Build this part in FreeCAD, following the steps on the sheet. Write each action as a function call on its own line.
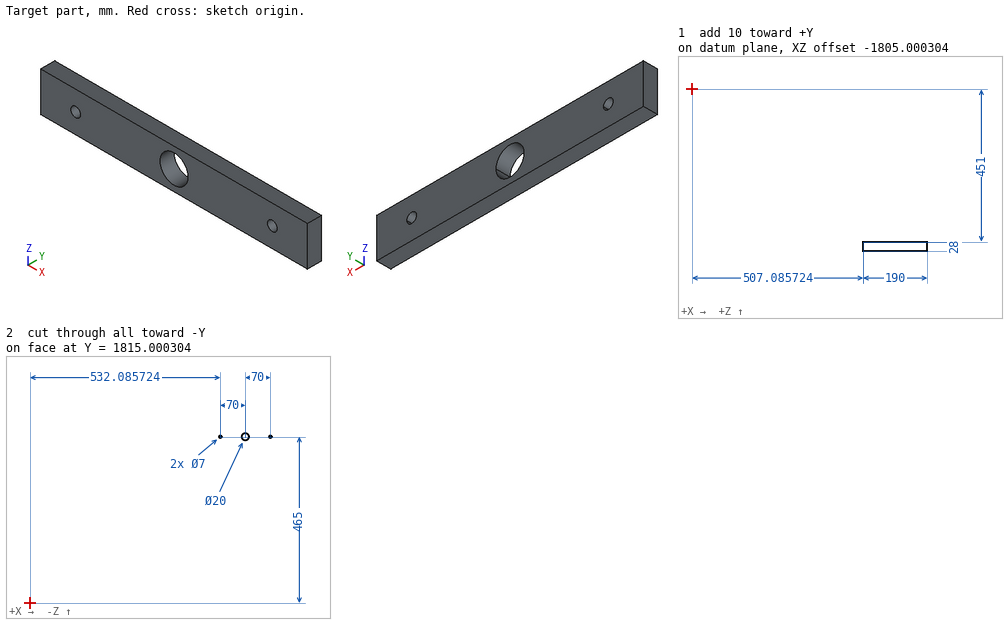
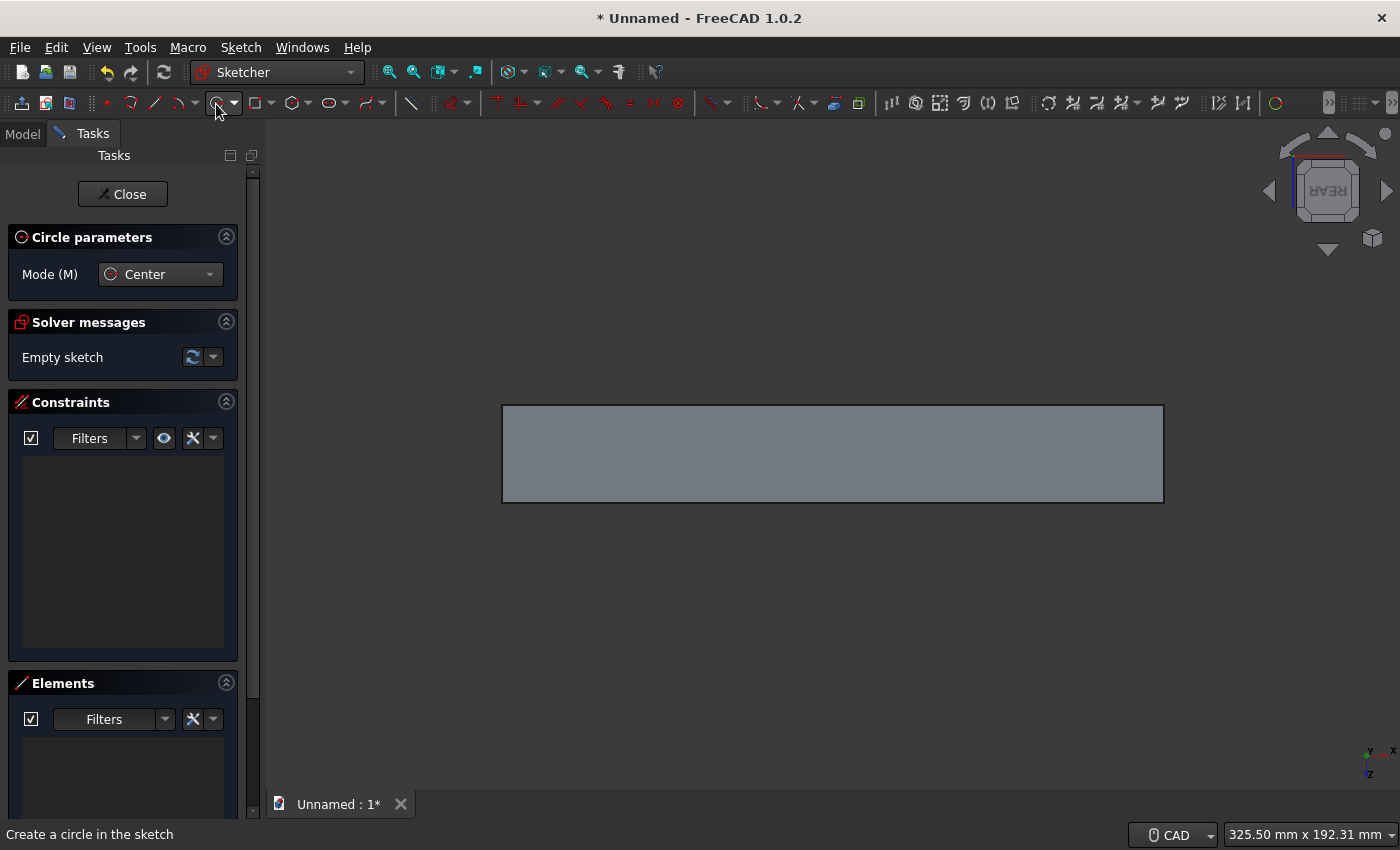
scroll(589, 454, up, 4)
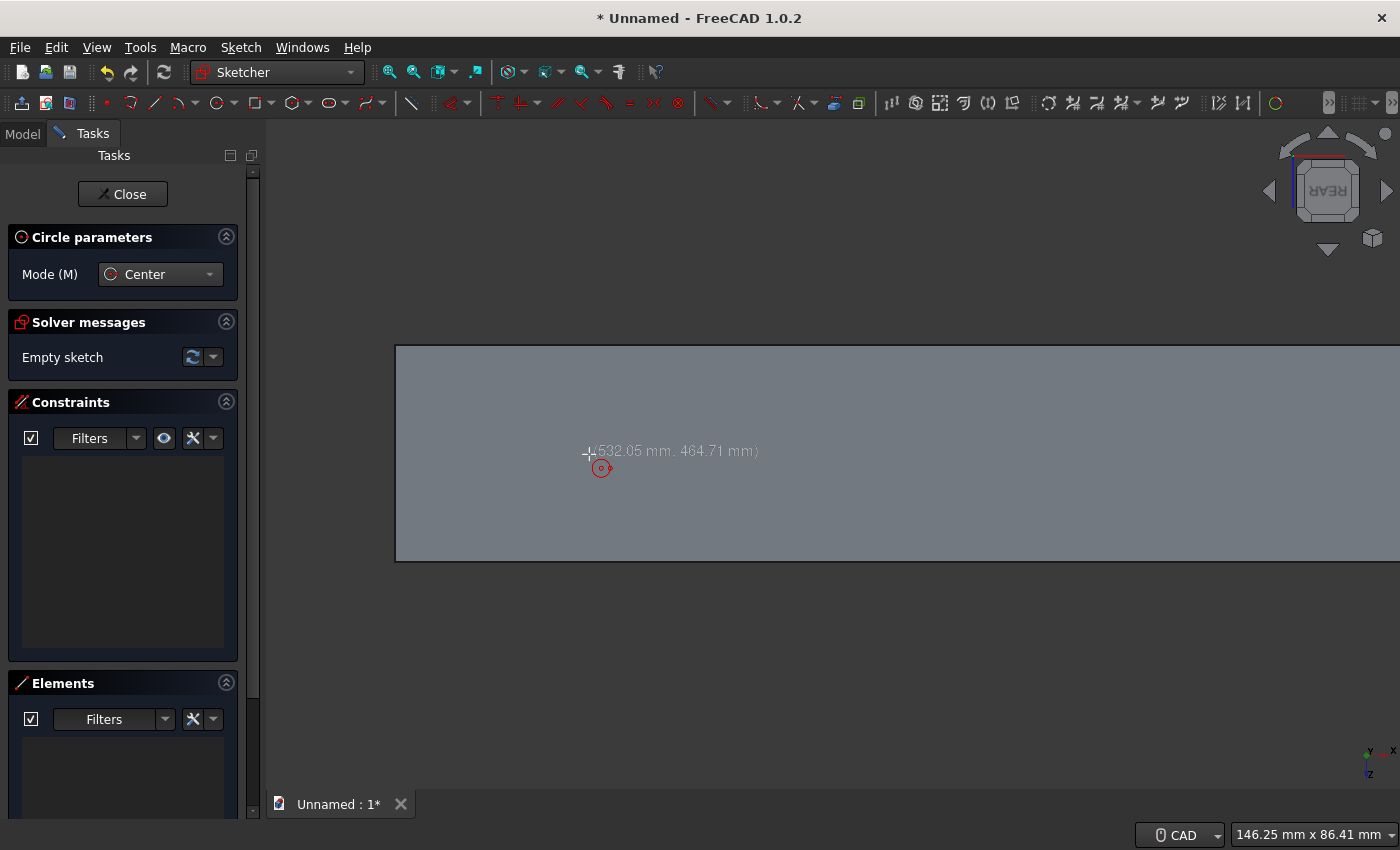
click(589, 453)
click(608, 434)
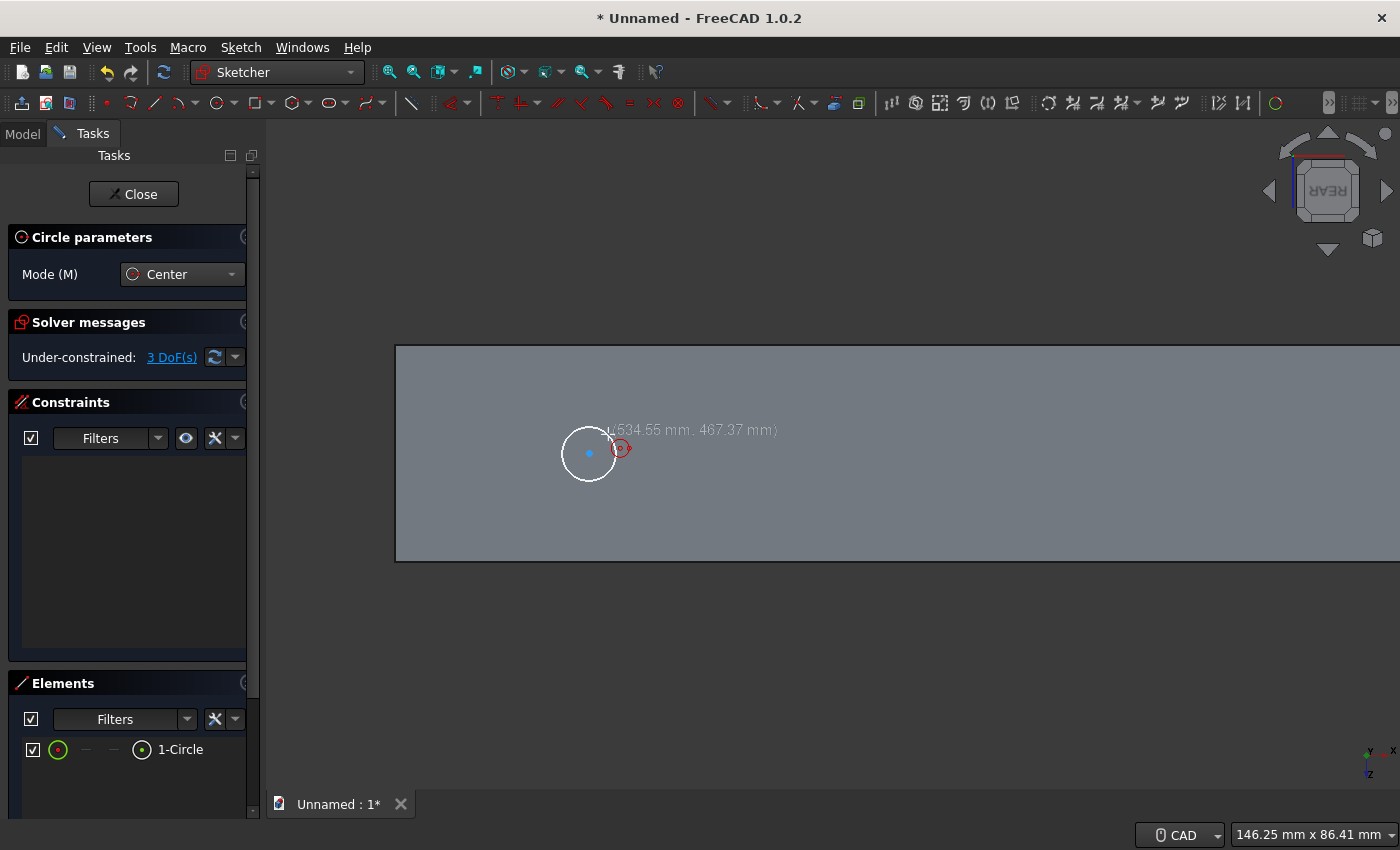
scroll(318, 455, down, 3)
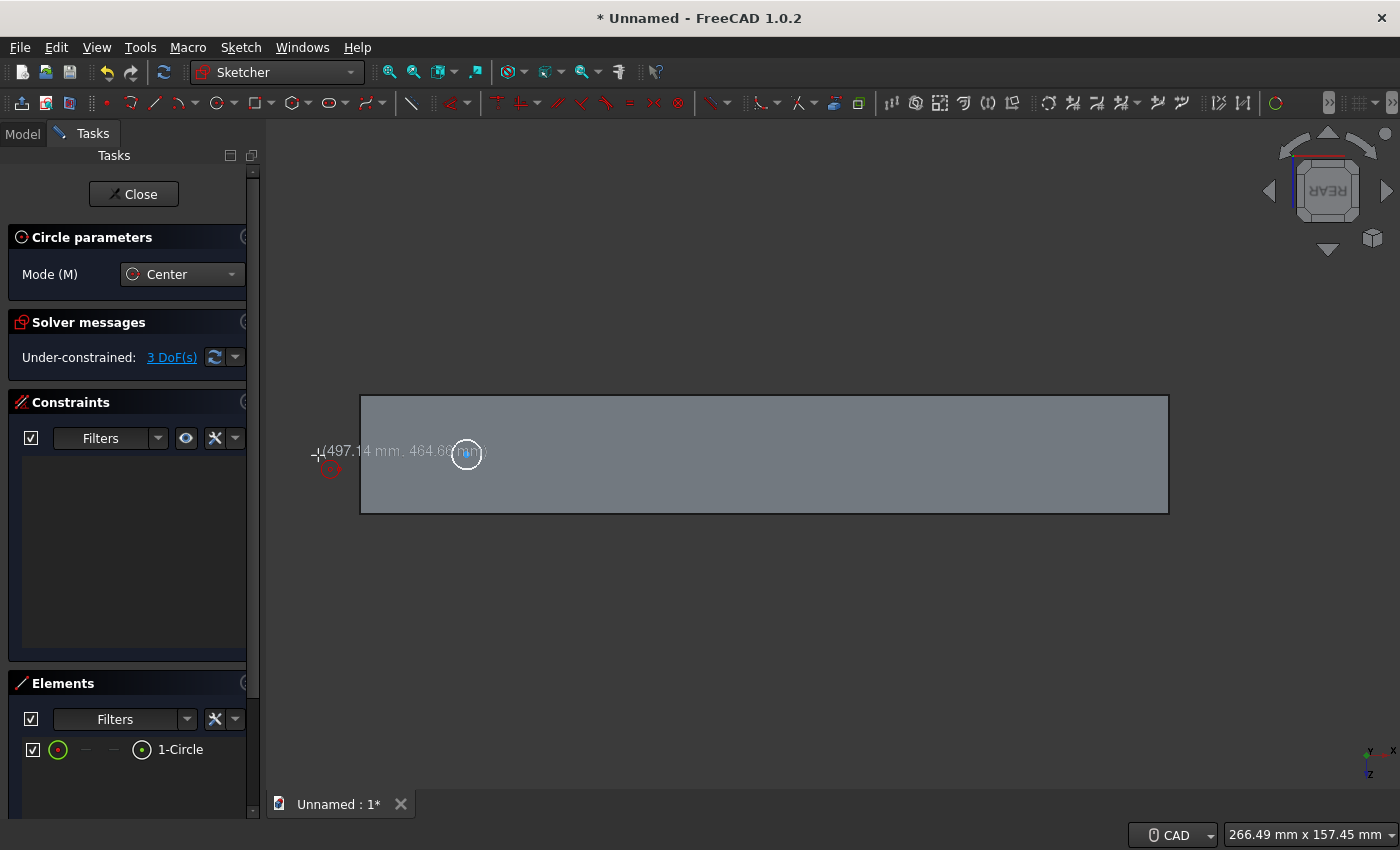
scroll(1062, 454, up, 3)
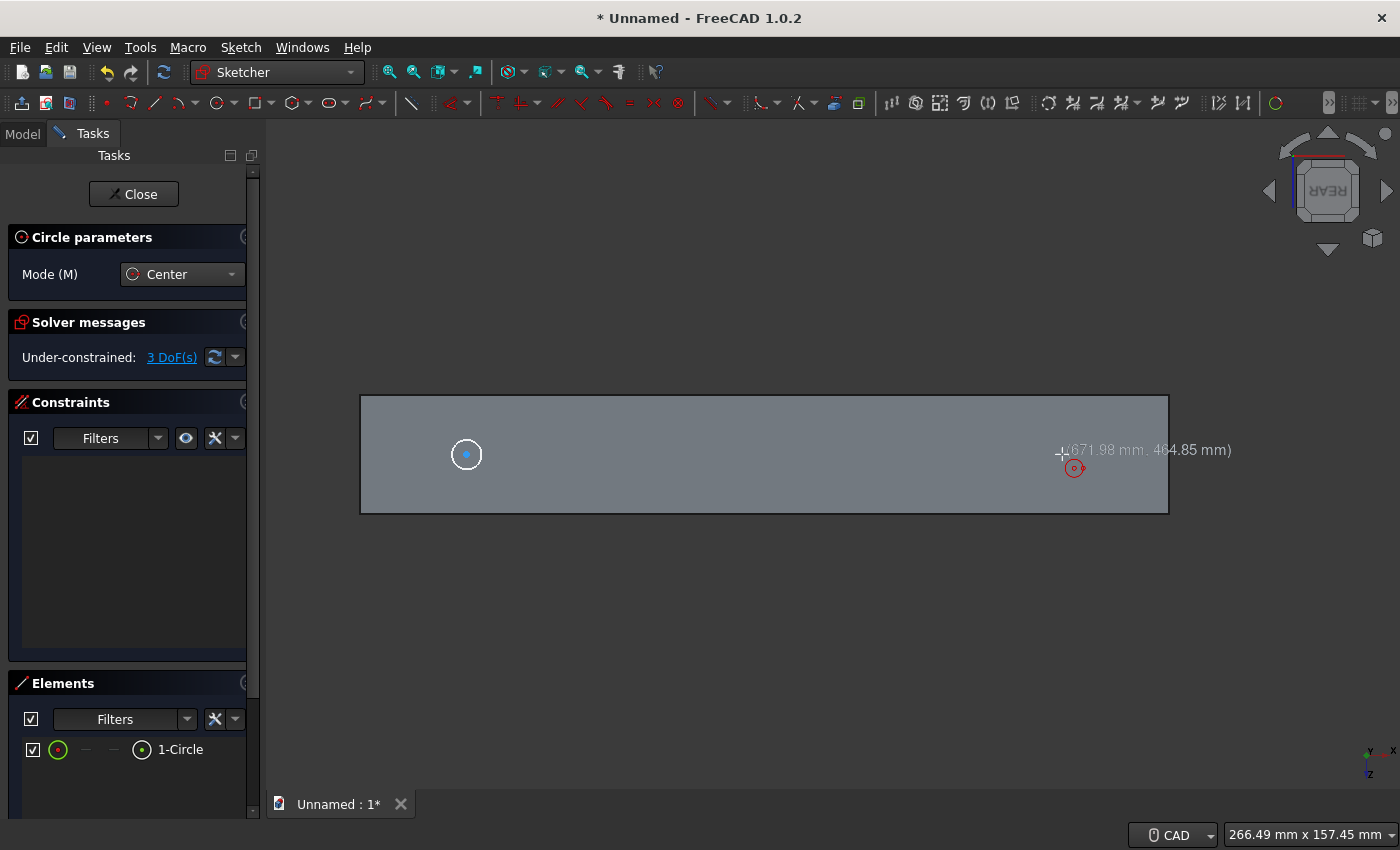
click(1062, 454)
click(1081, 435)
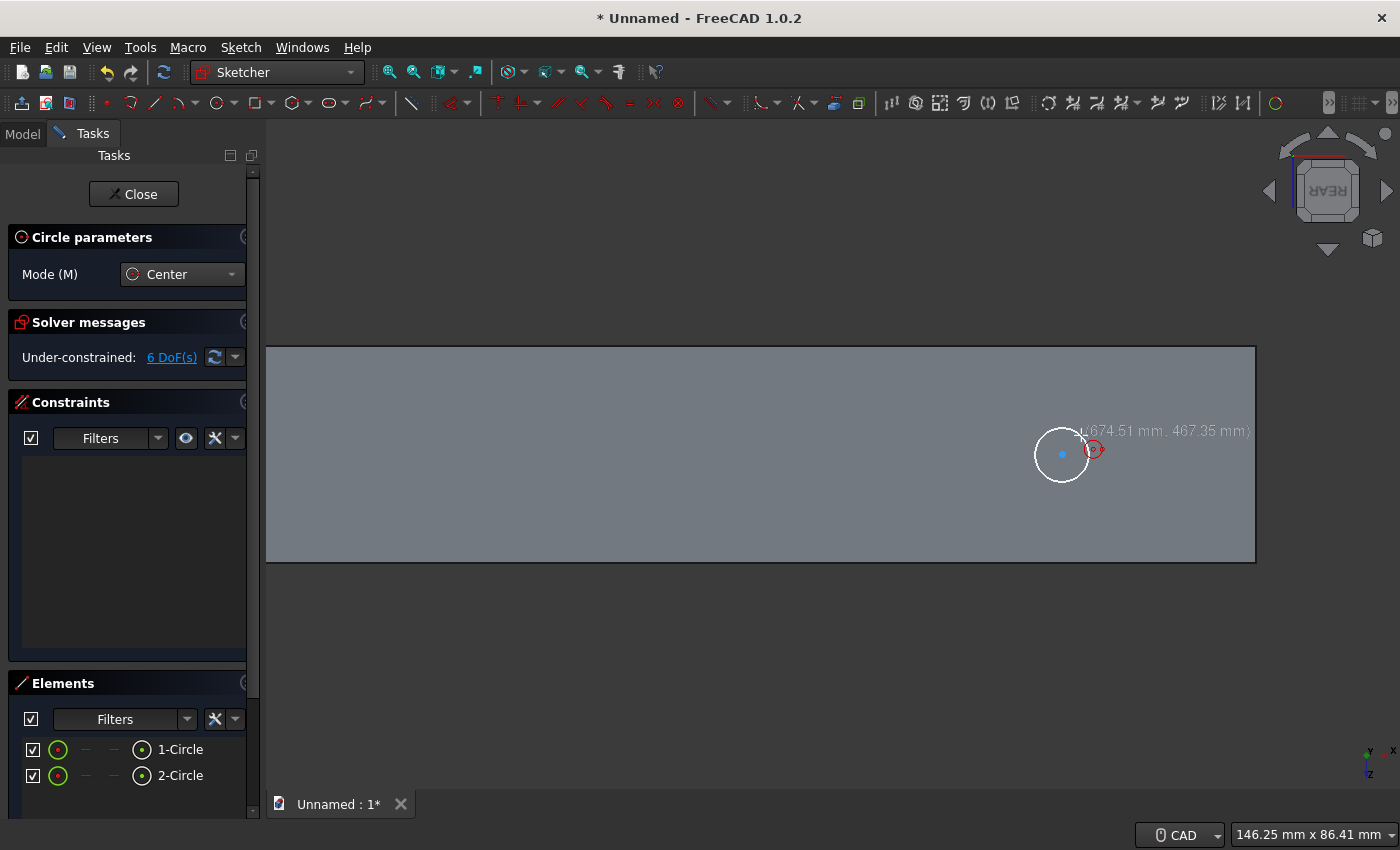
click(519, 454)
click(574, 399)
key(Escape)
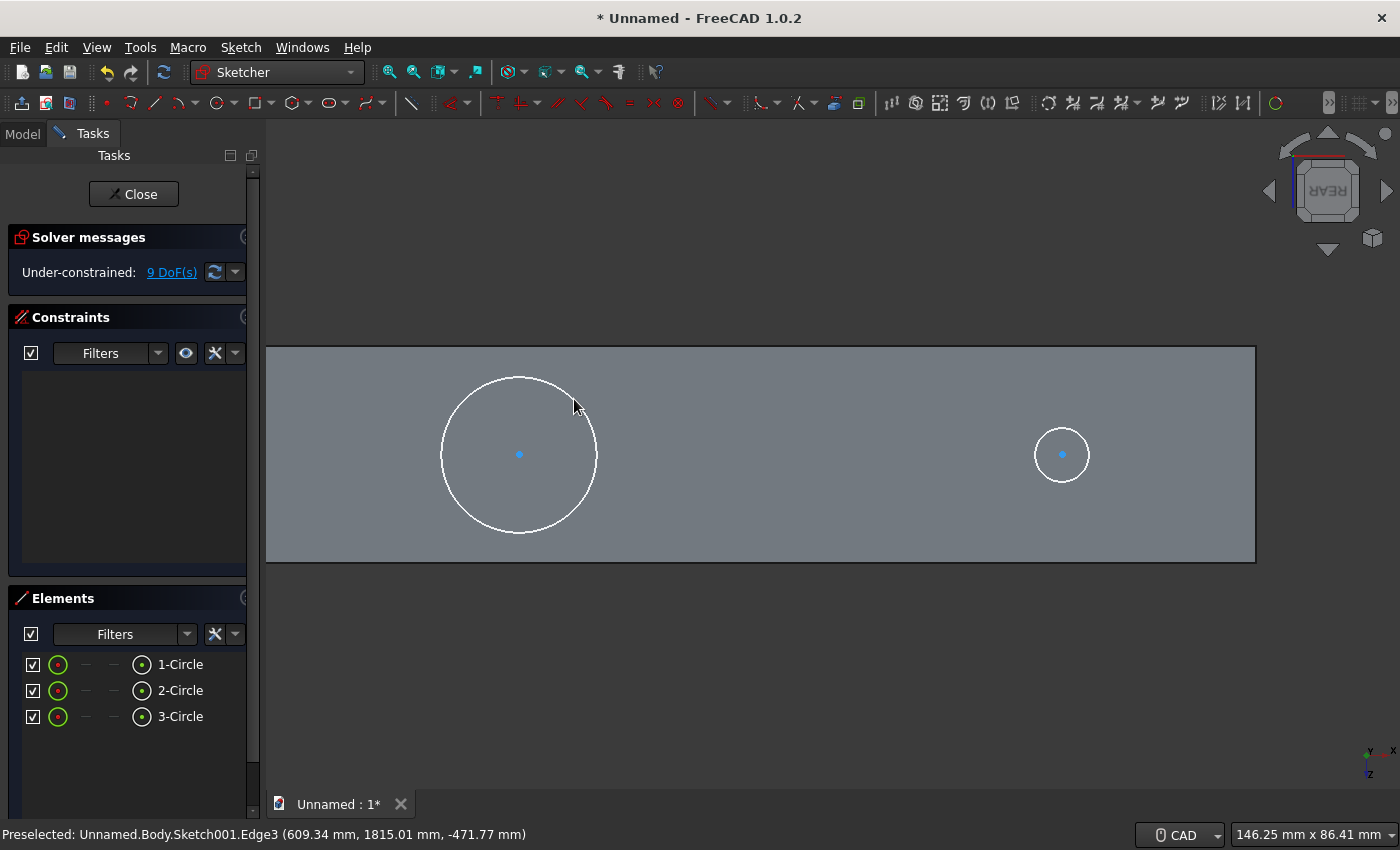
scroll(1063, 454, down, 3)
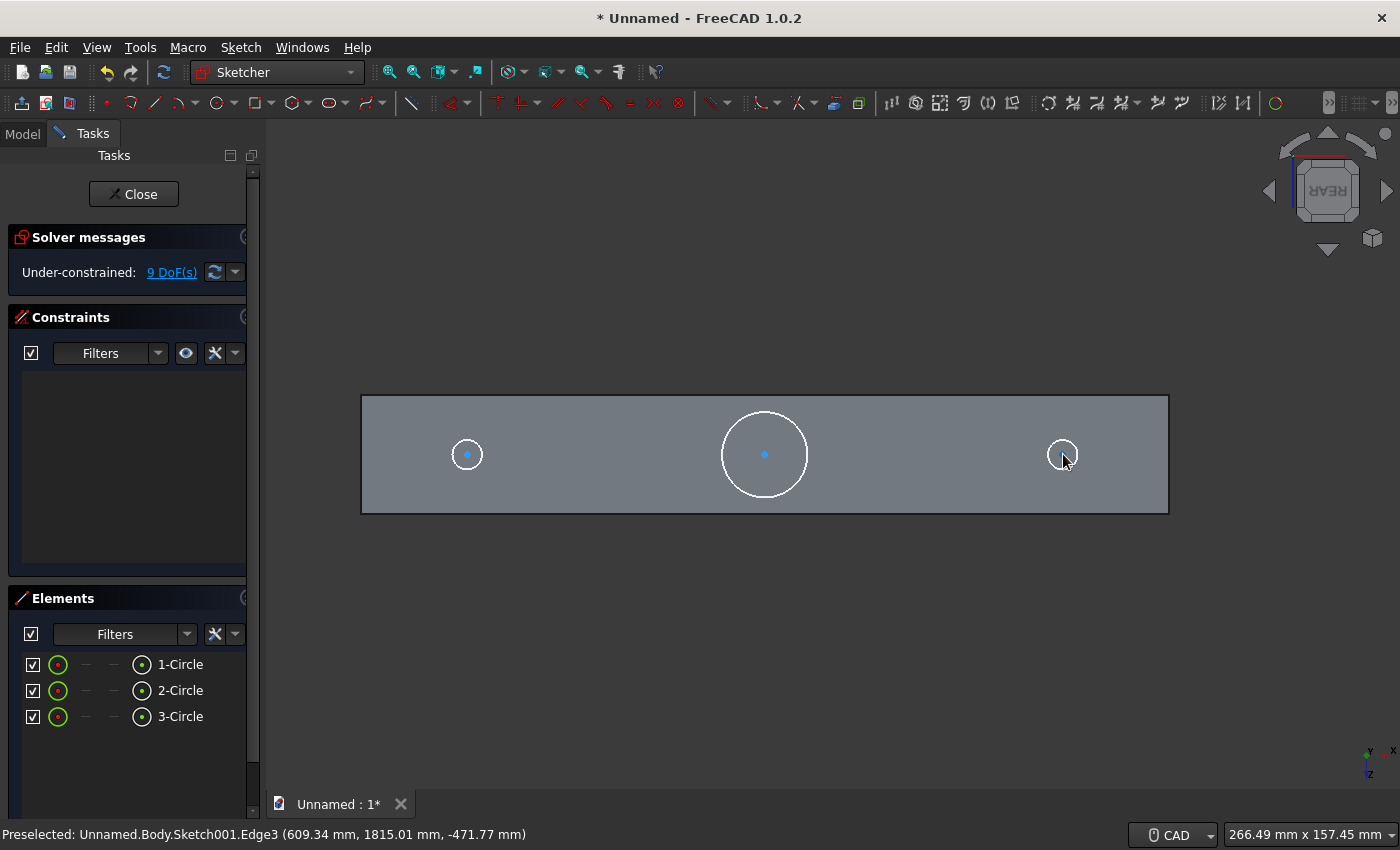
click(478, 444)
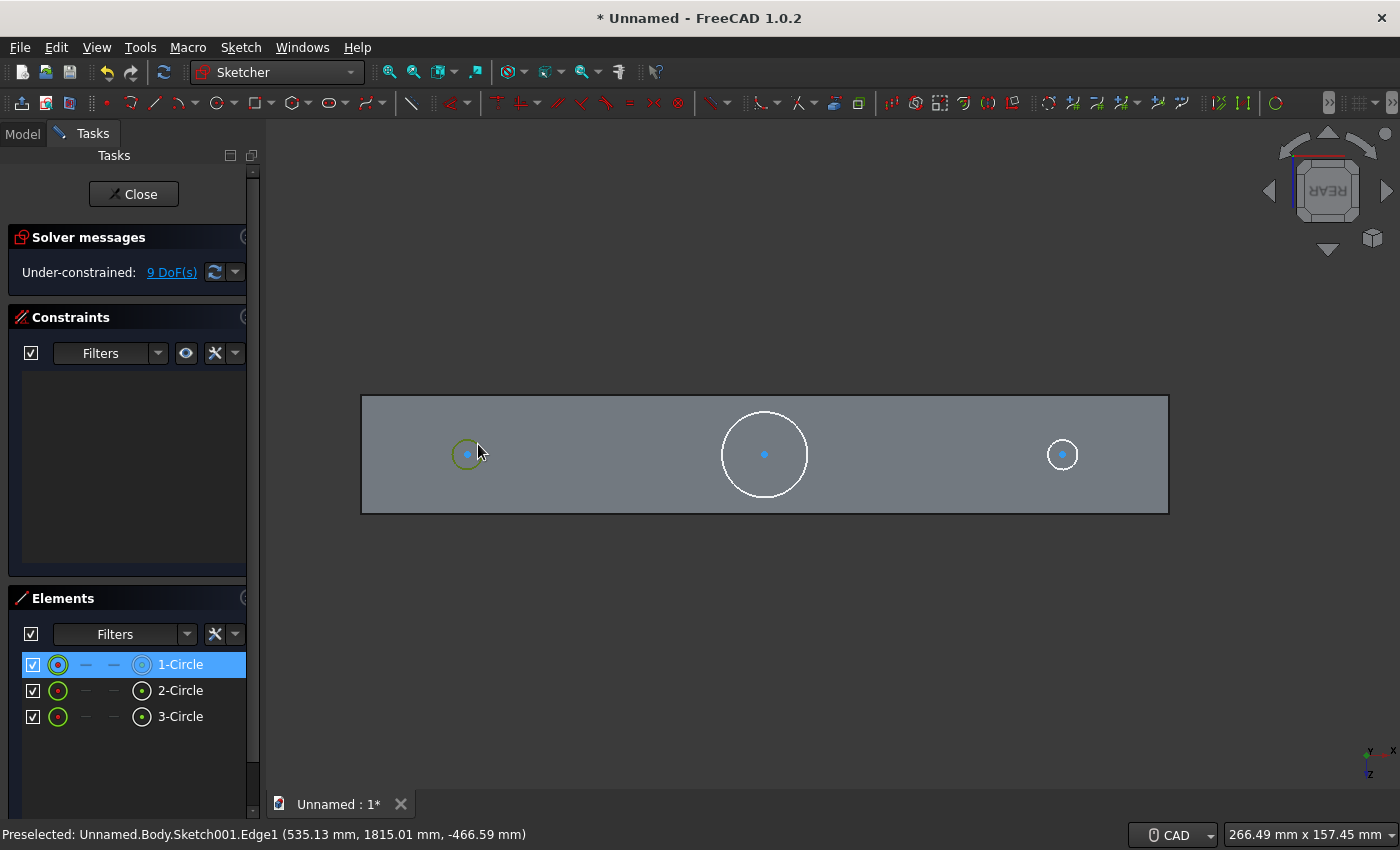
click(1073, 444)